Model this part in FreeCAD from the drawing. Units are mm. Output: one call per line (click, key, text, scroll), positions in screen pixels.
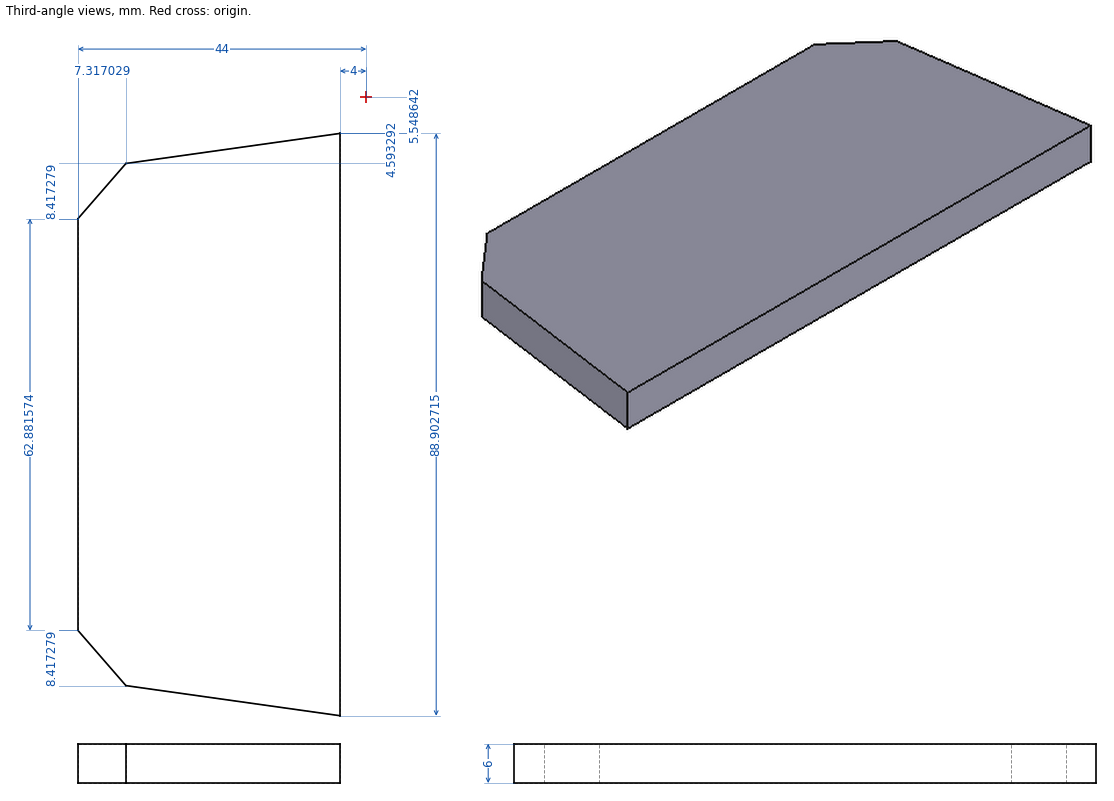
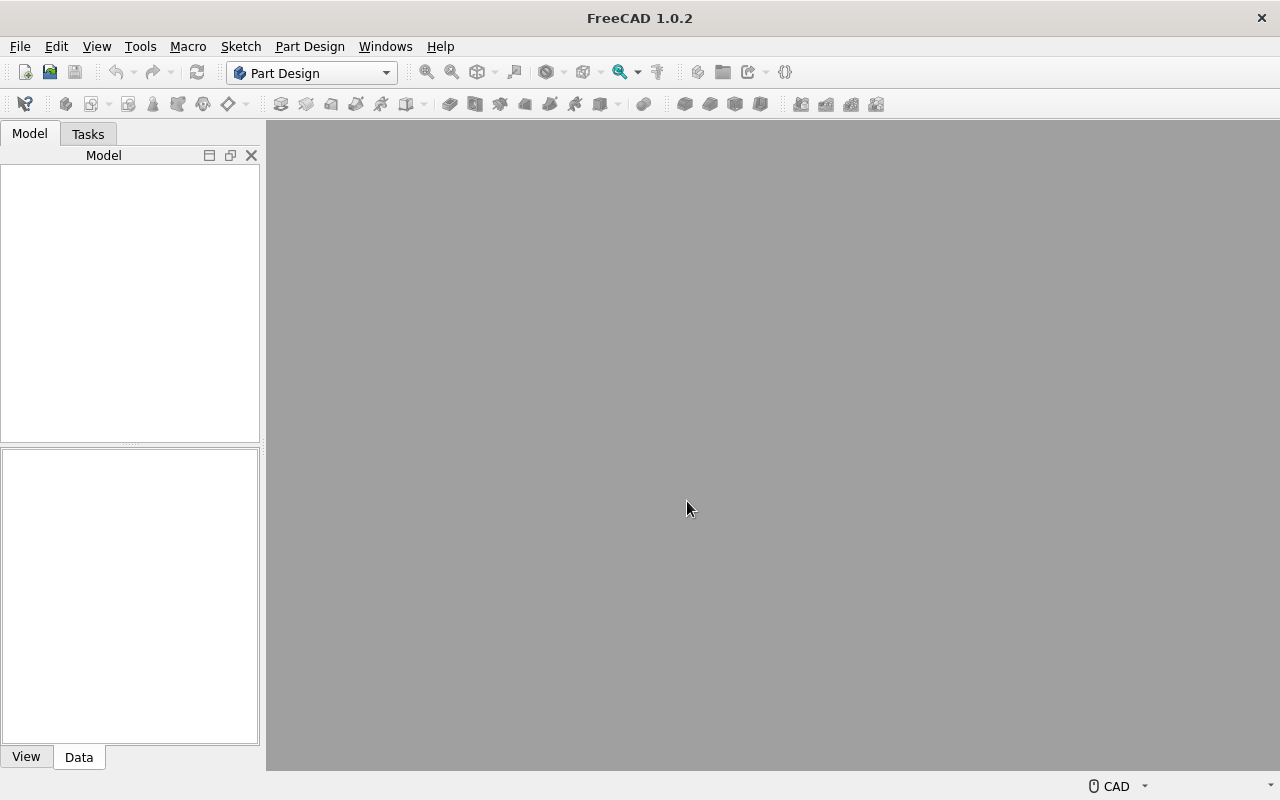
click(25, 72)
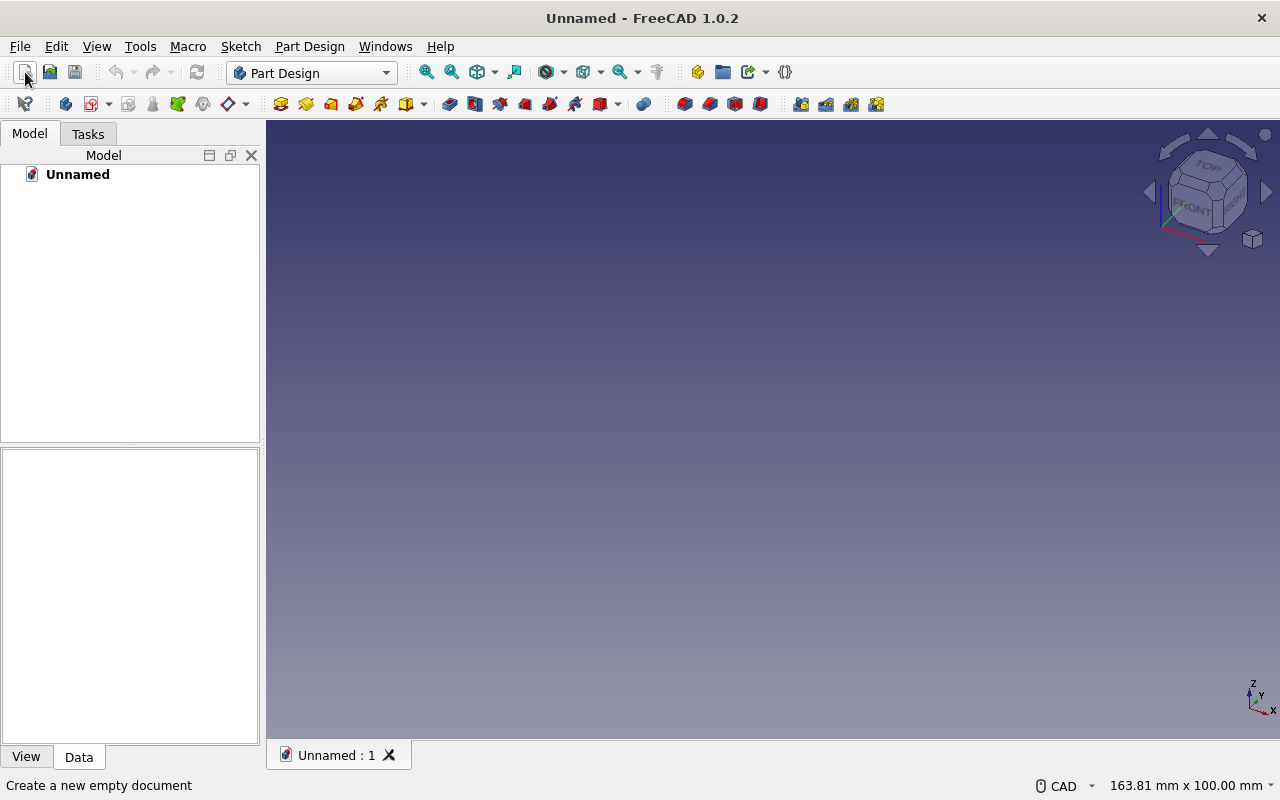
click(90, 104)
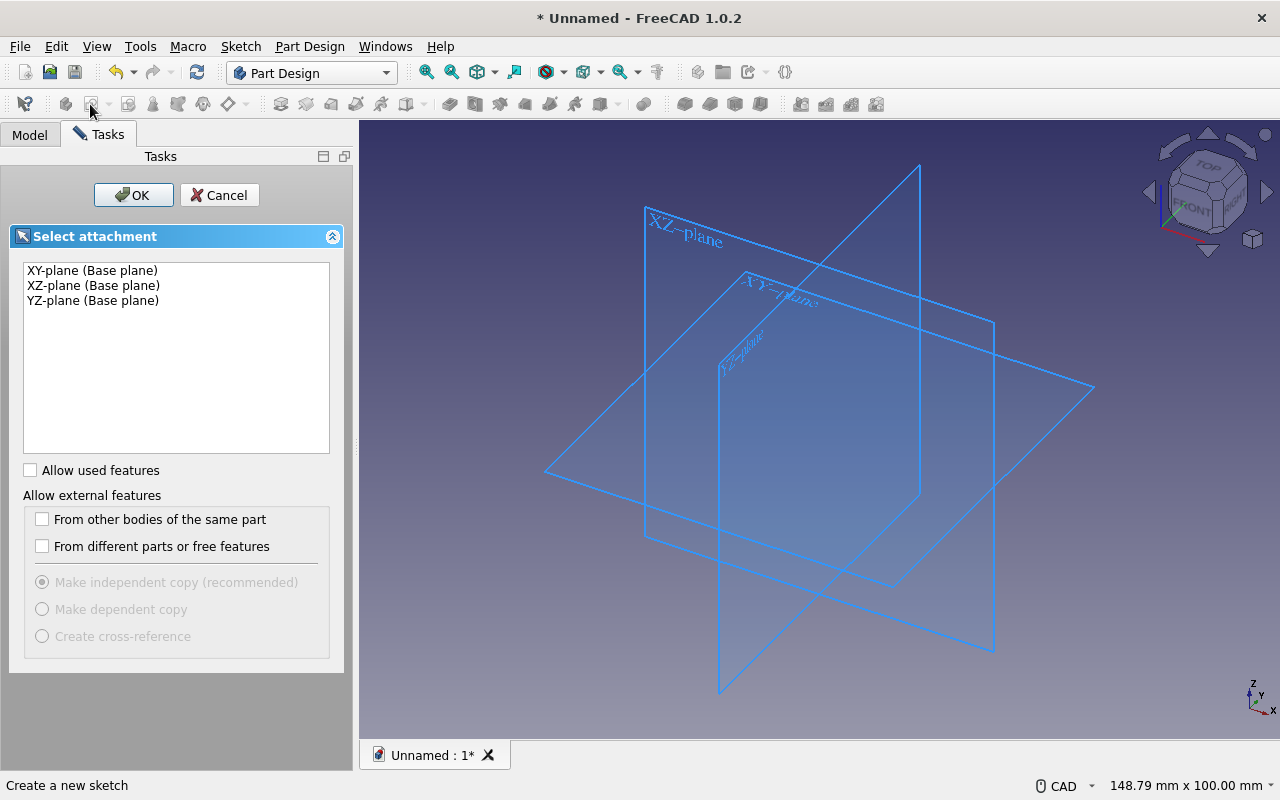
click(84, 270)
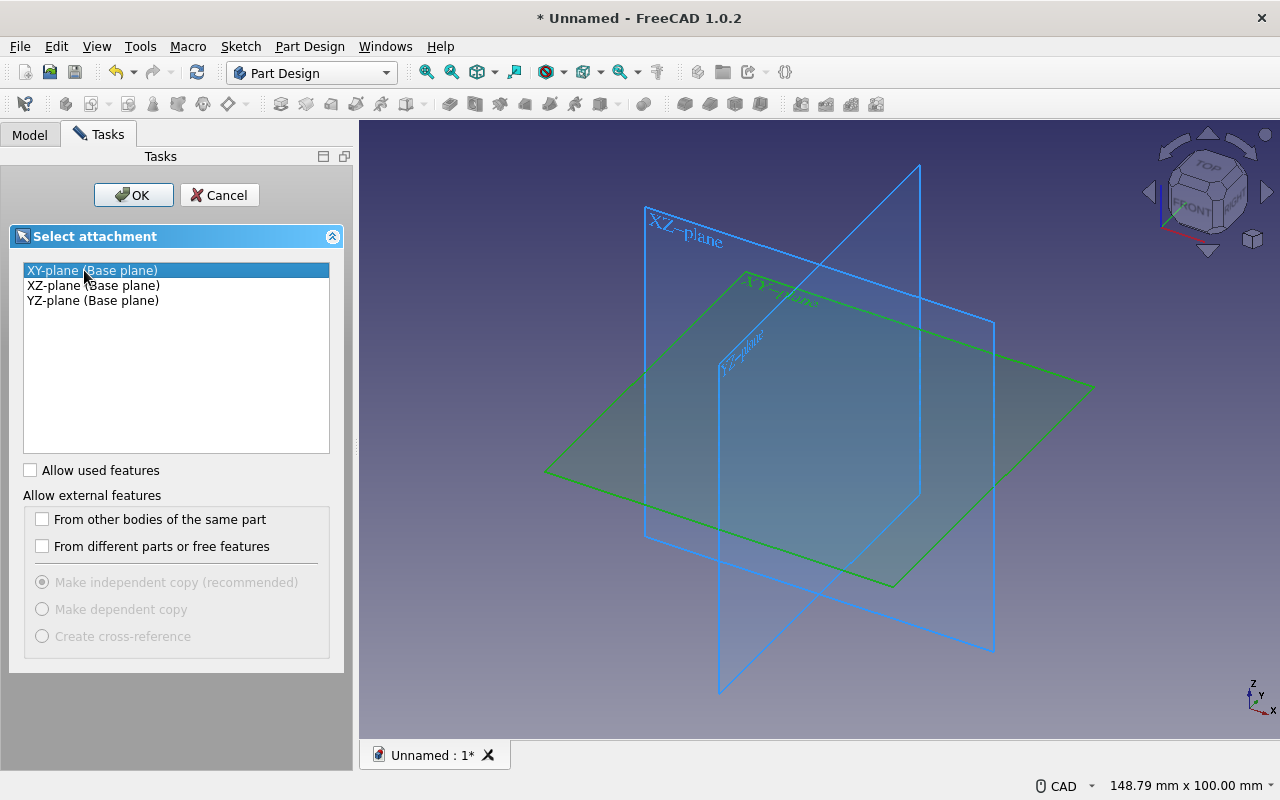
click(134, 195)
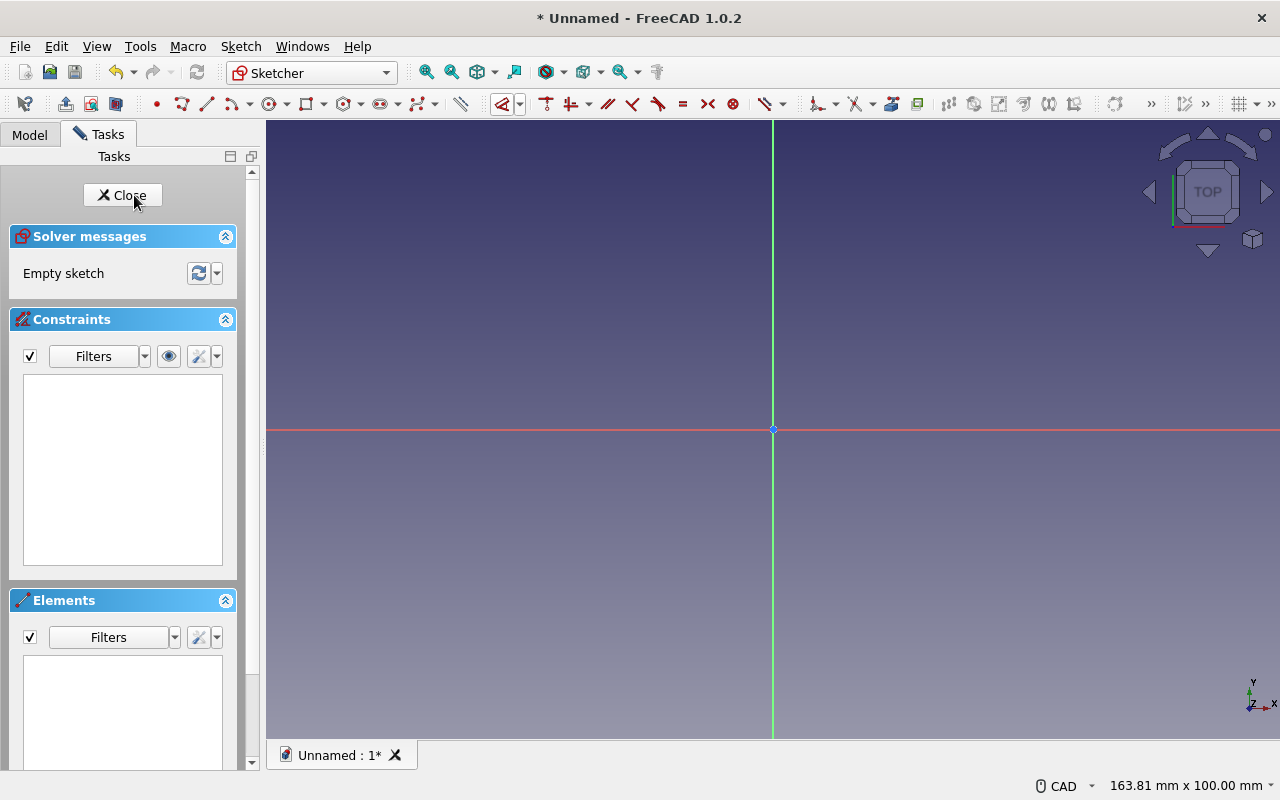
scroll(787, 148, down, 3)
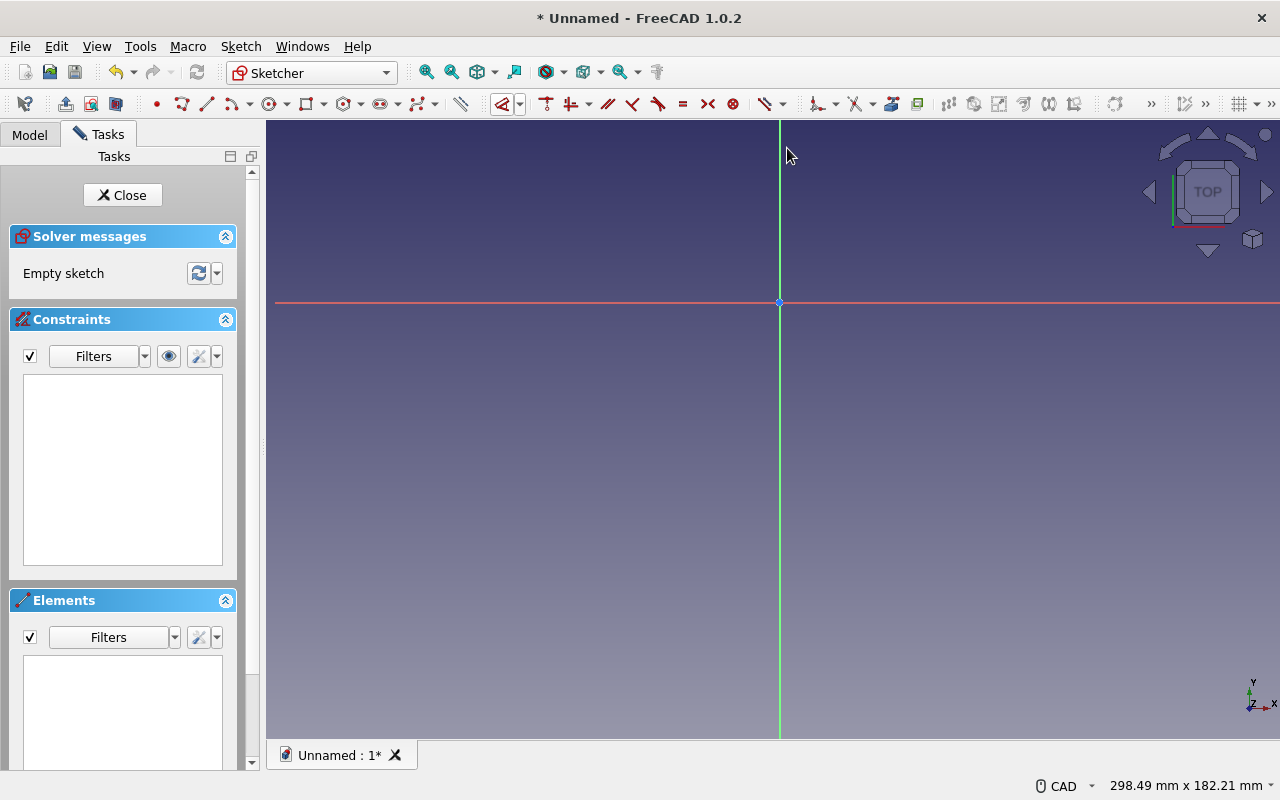
click(182, 104)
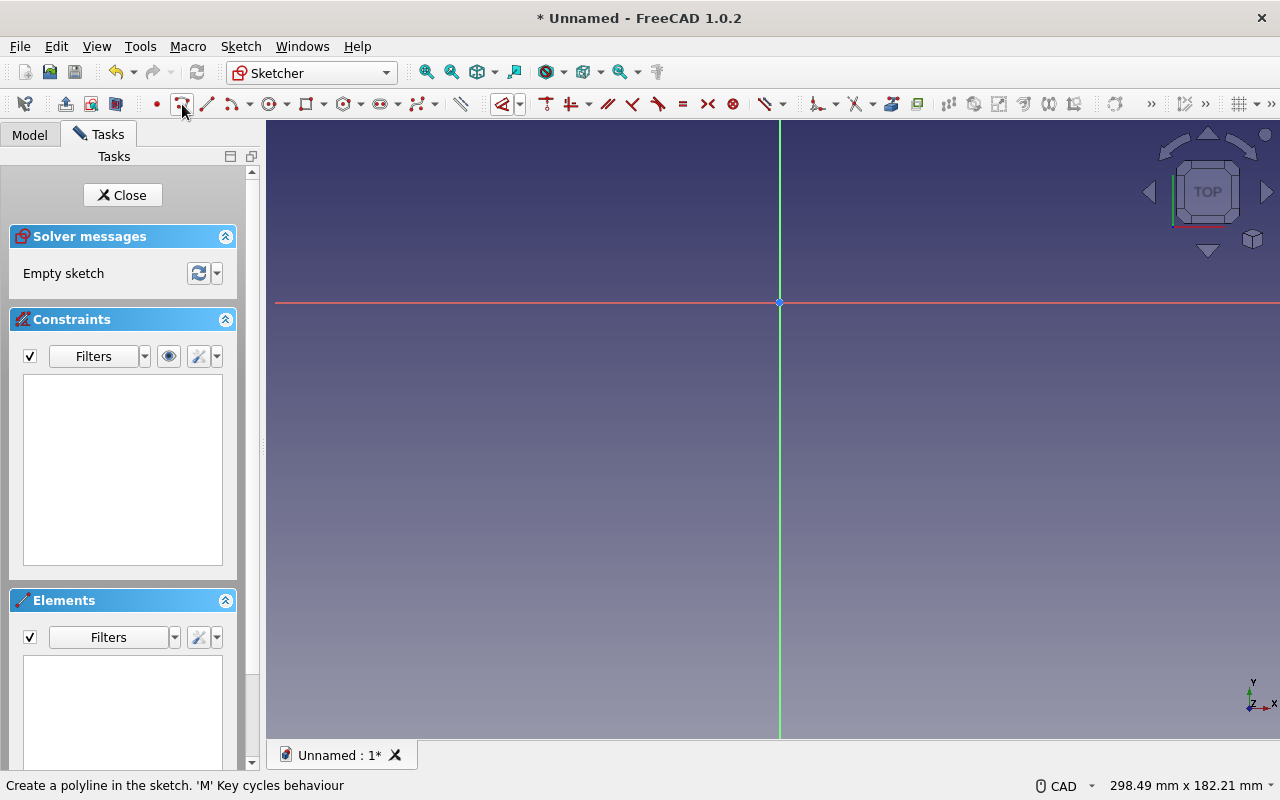
click(766, 321)
click(655, 337)
click(630, 366)
click(630, 579)
click(655, 608)
click(766, 623)
click(766, 322)
key(Escape)
key(Escape)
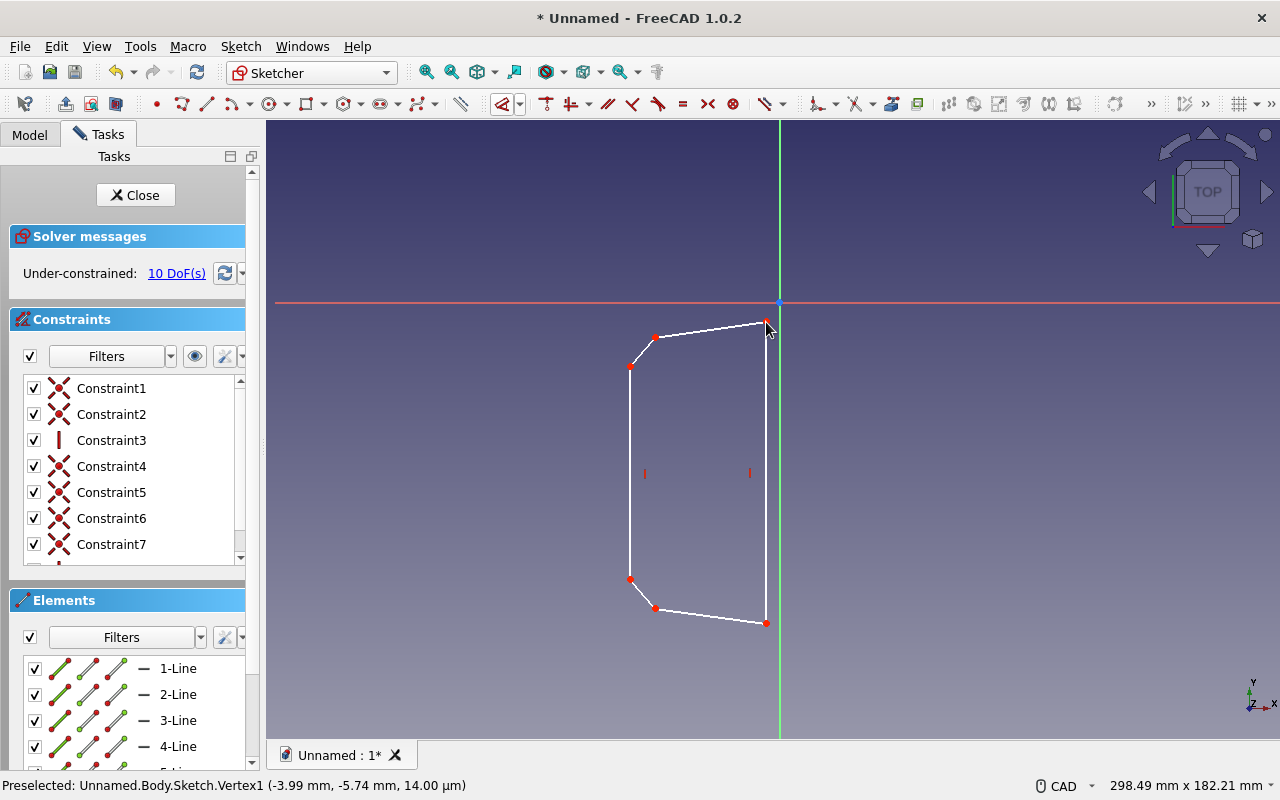
click(502, 104)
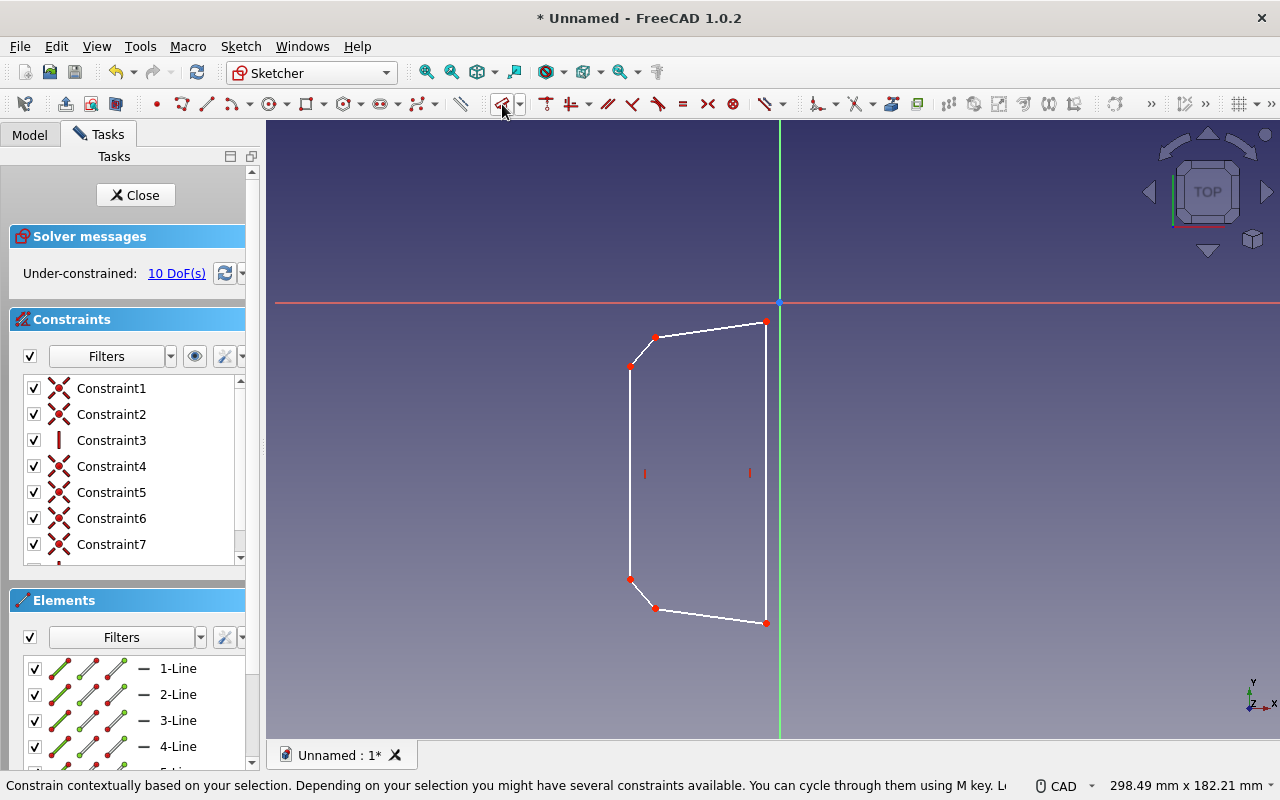
scroll(766, 322, up, 6)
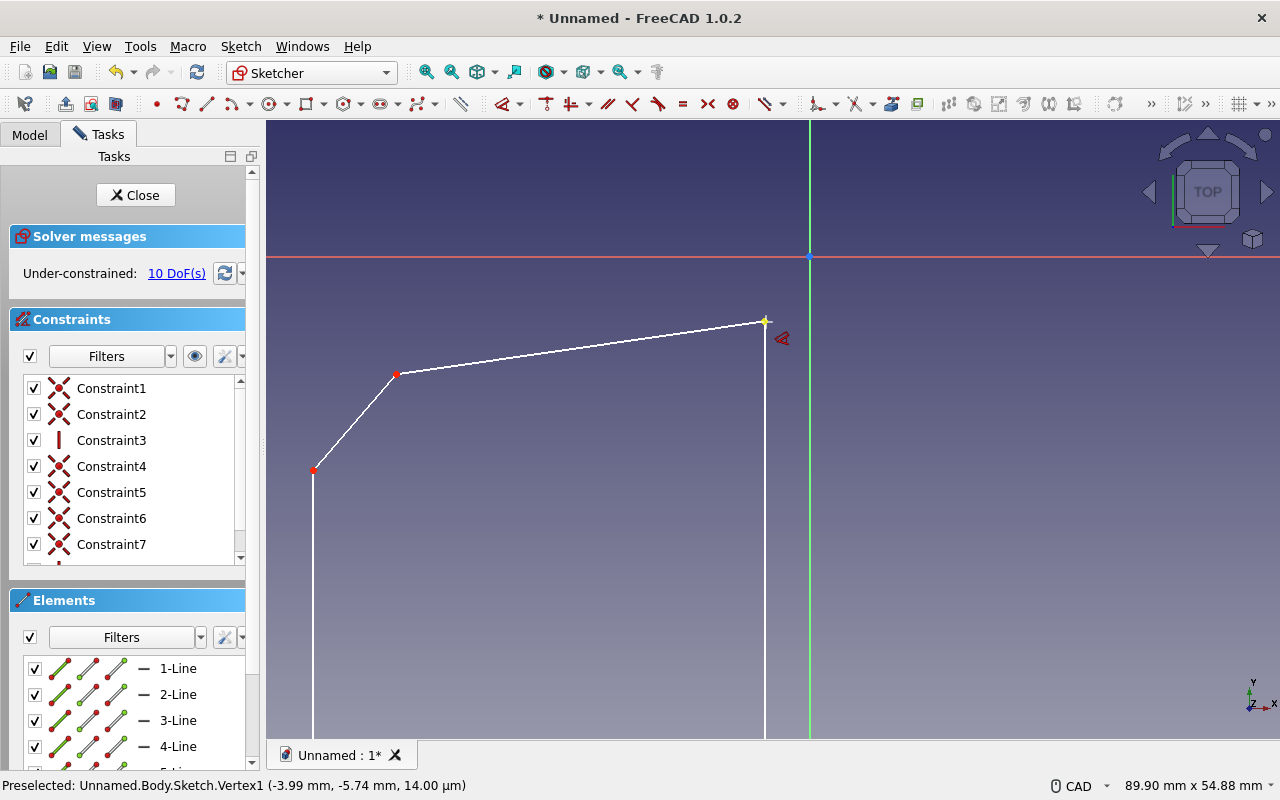
click(765, 321)
click(787, 223)